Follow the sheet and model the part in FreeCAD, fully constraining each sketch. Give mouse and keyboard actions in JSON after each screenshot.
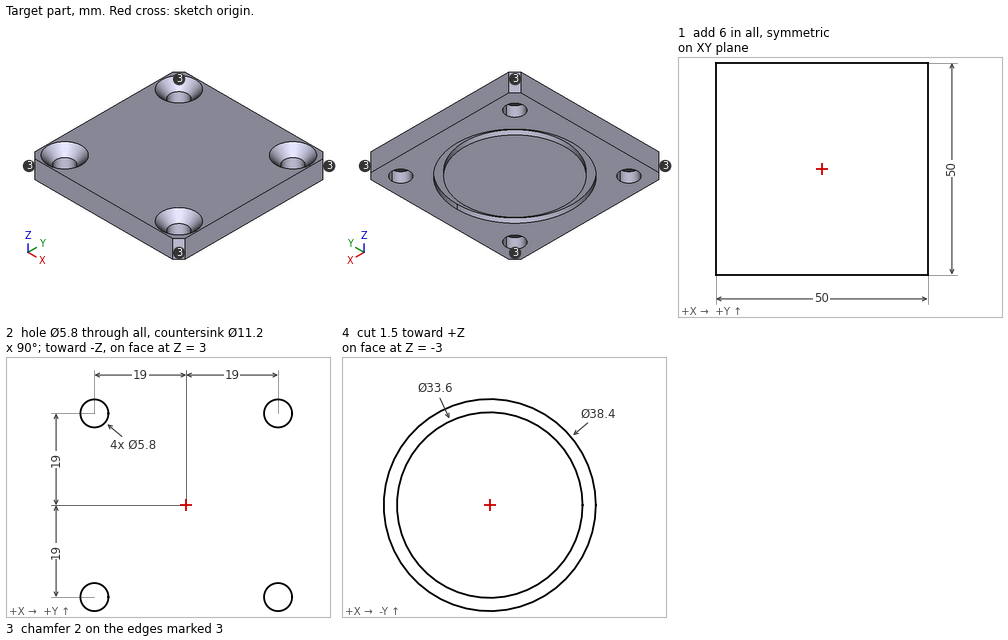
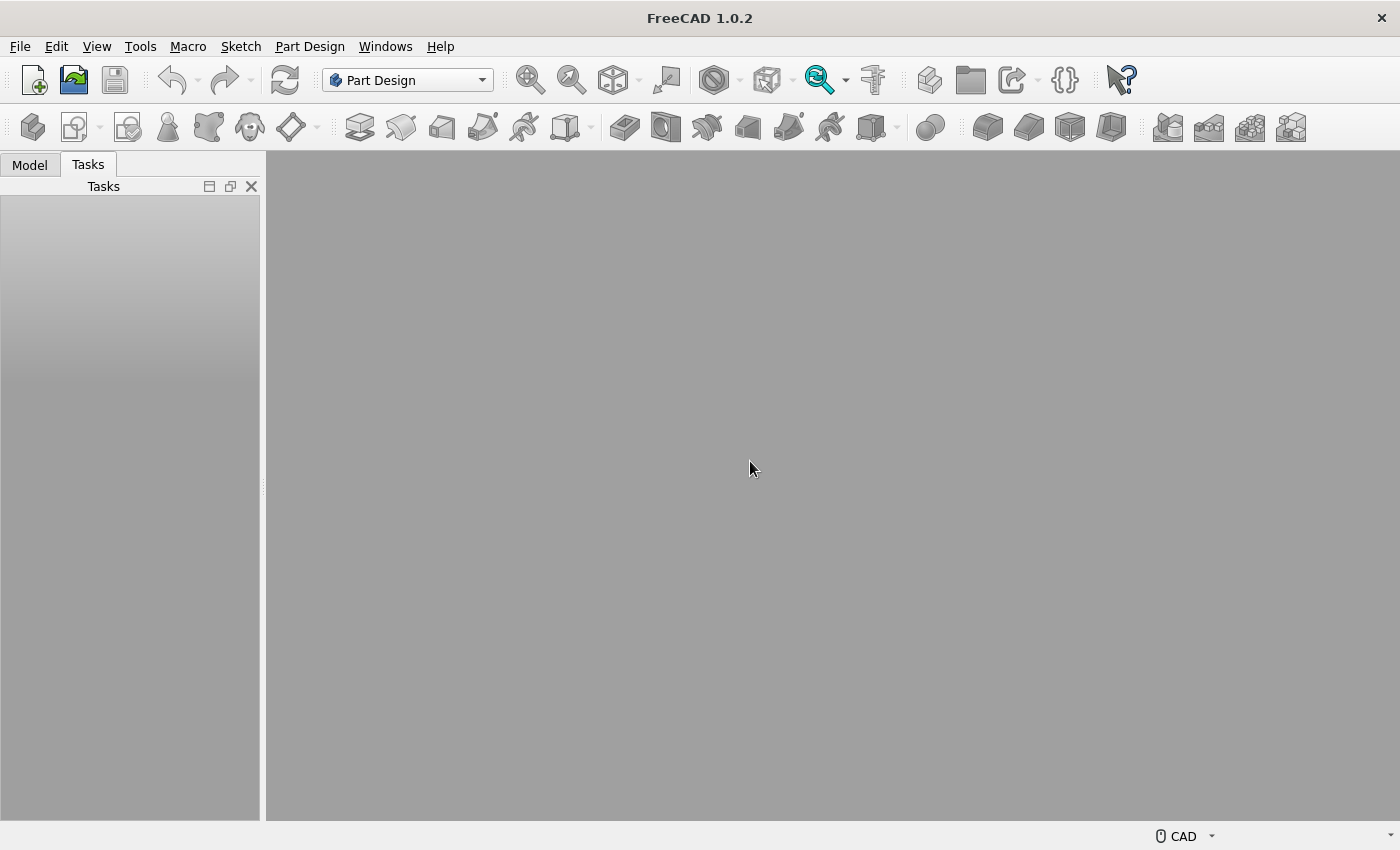
{"action": "left_click", "coordinate": [33, 80]}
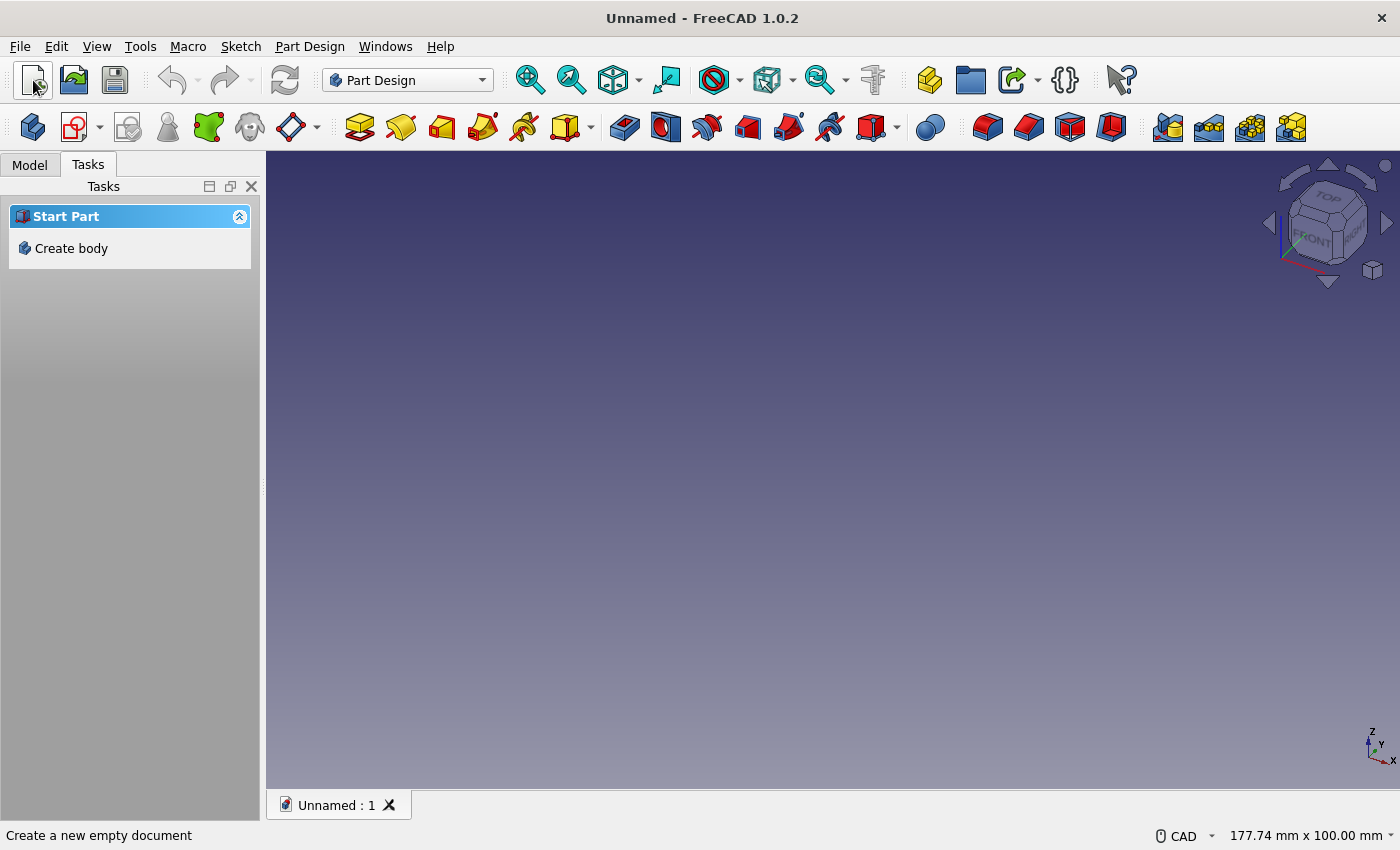
{"action": "left_click", "coordinate": [74, 128]}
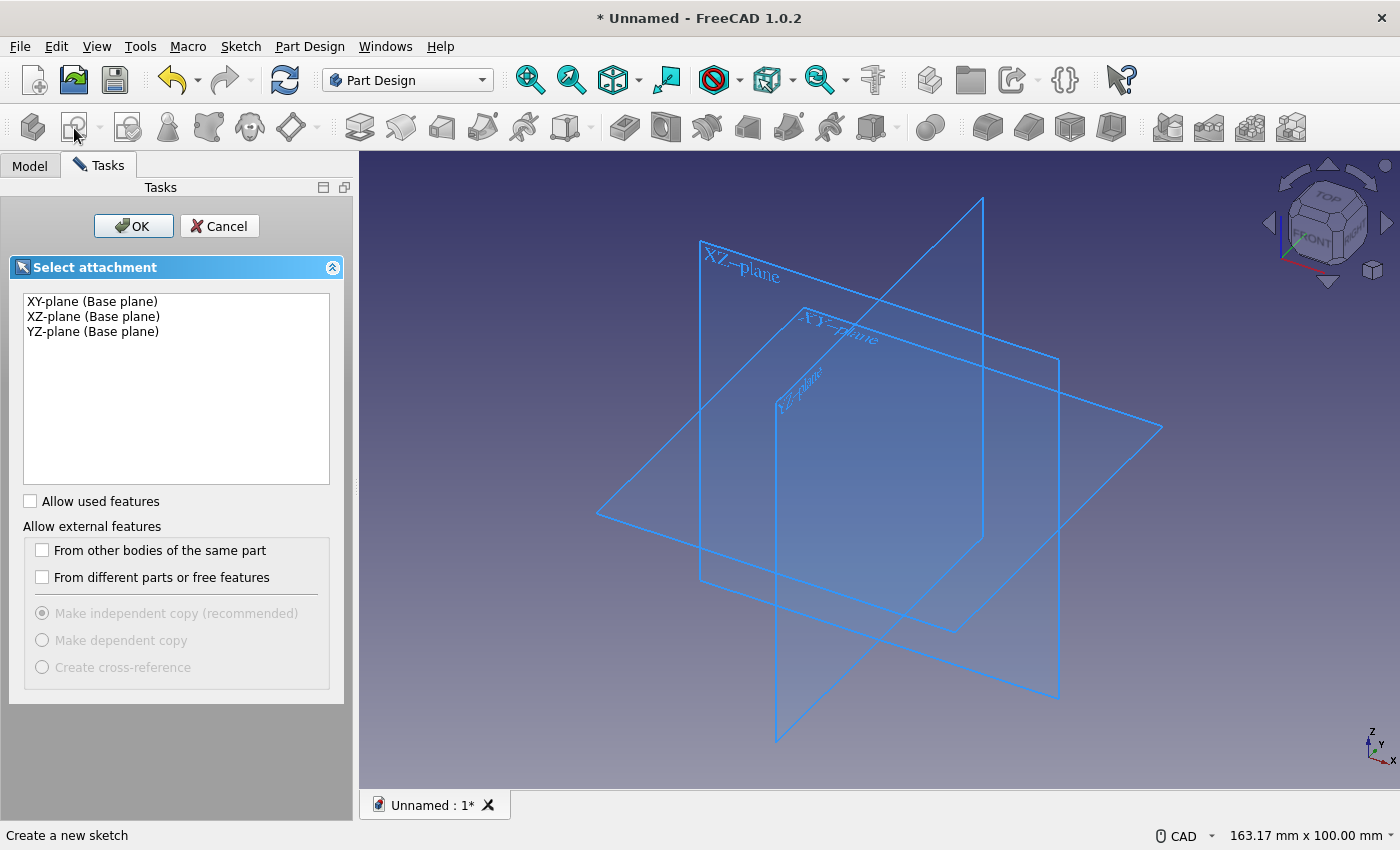
{"action": "left_click", "coordinate": [84, 302]}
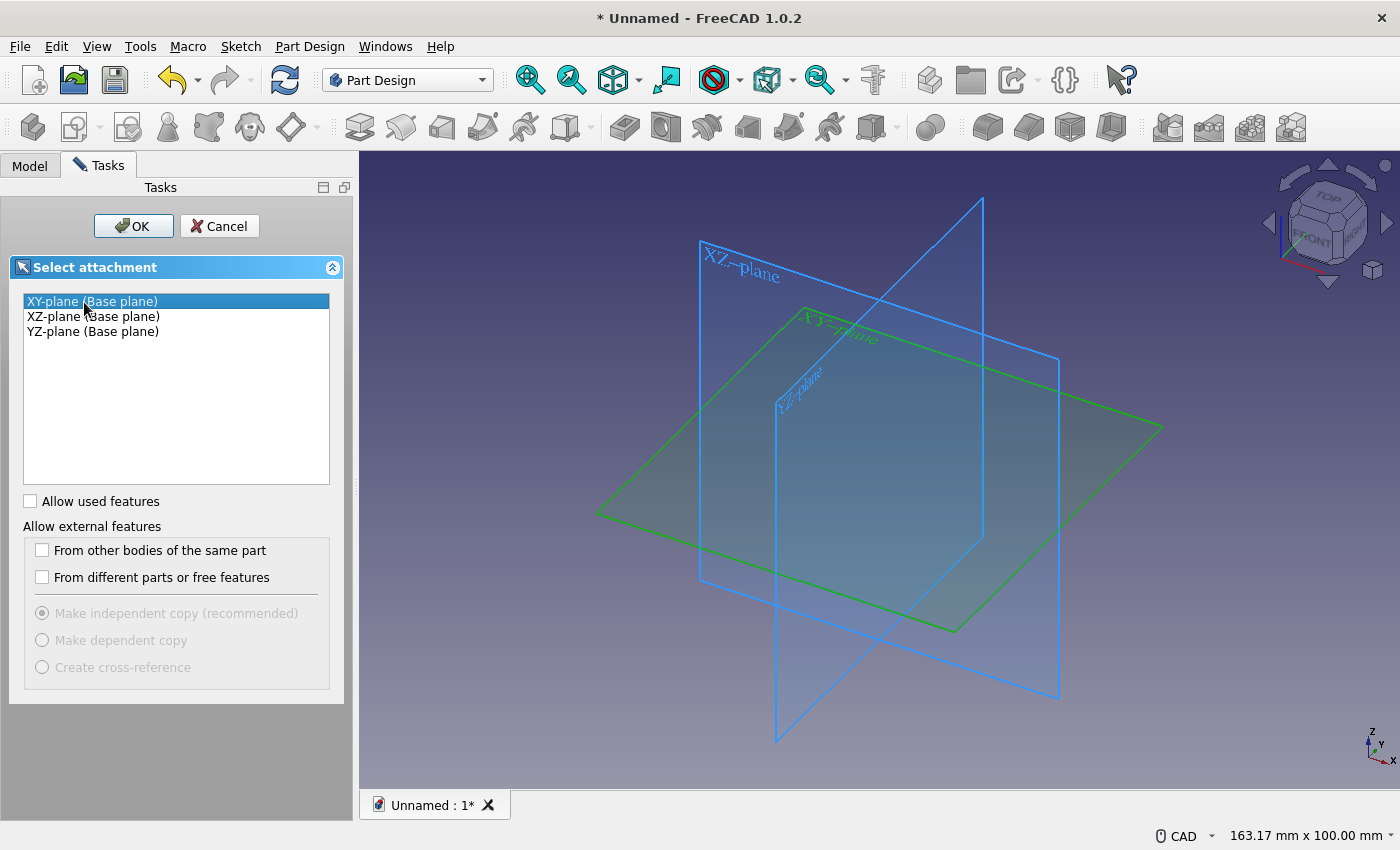
{"action": "left_click", "coordinate": [134, 226]}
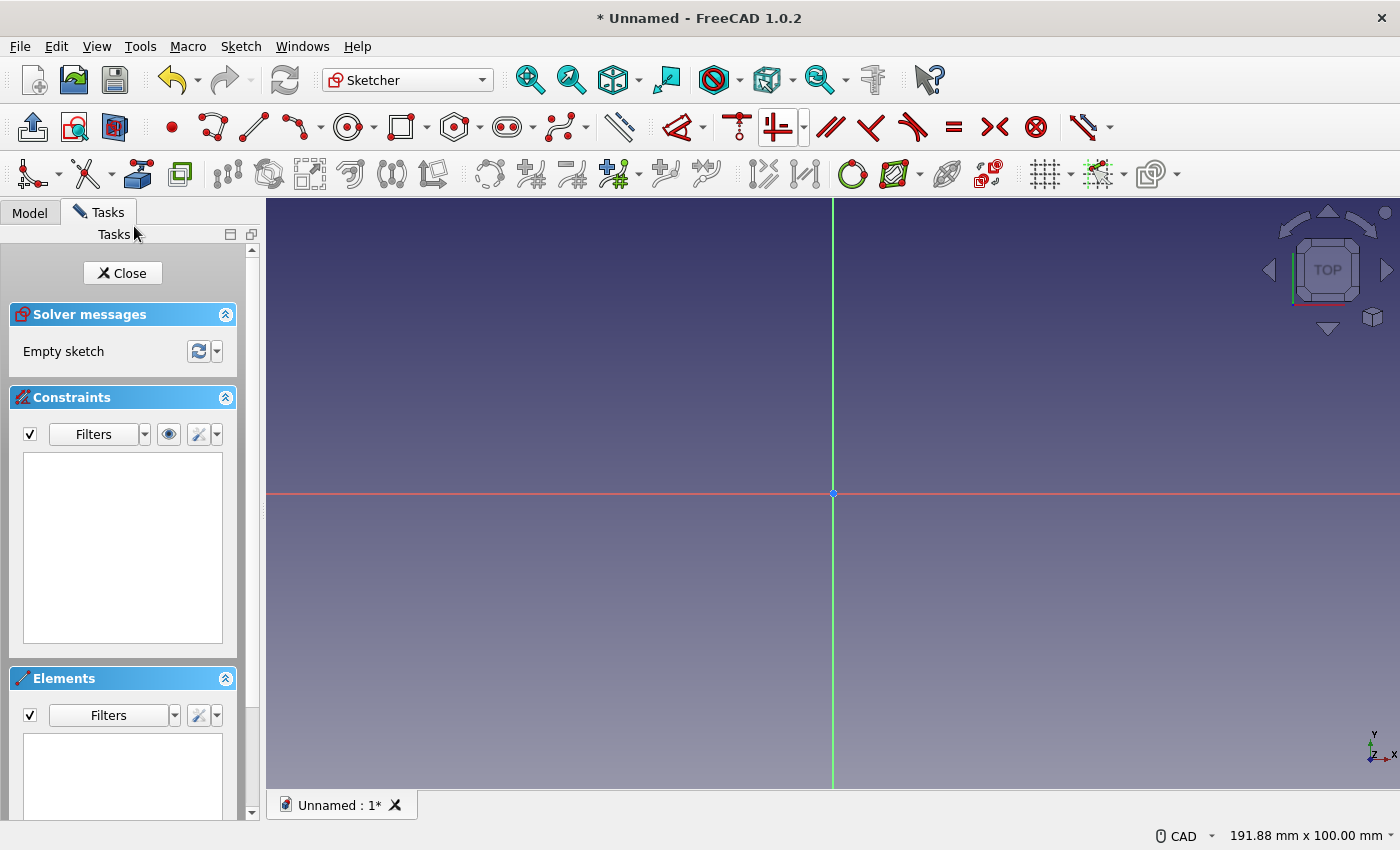
{"action": "left_click", "coordinate": [426, 128]}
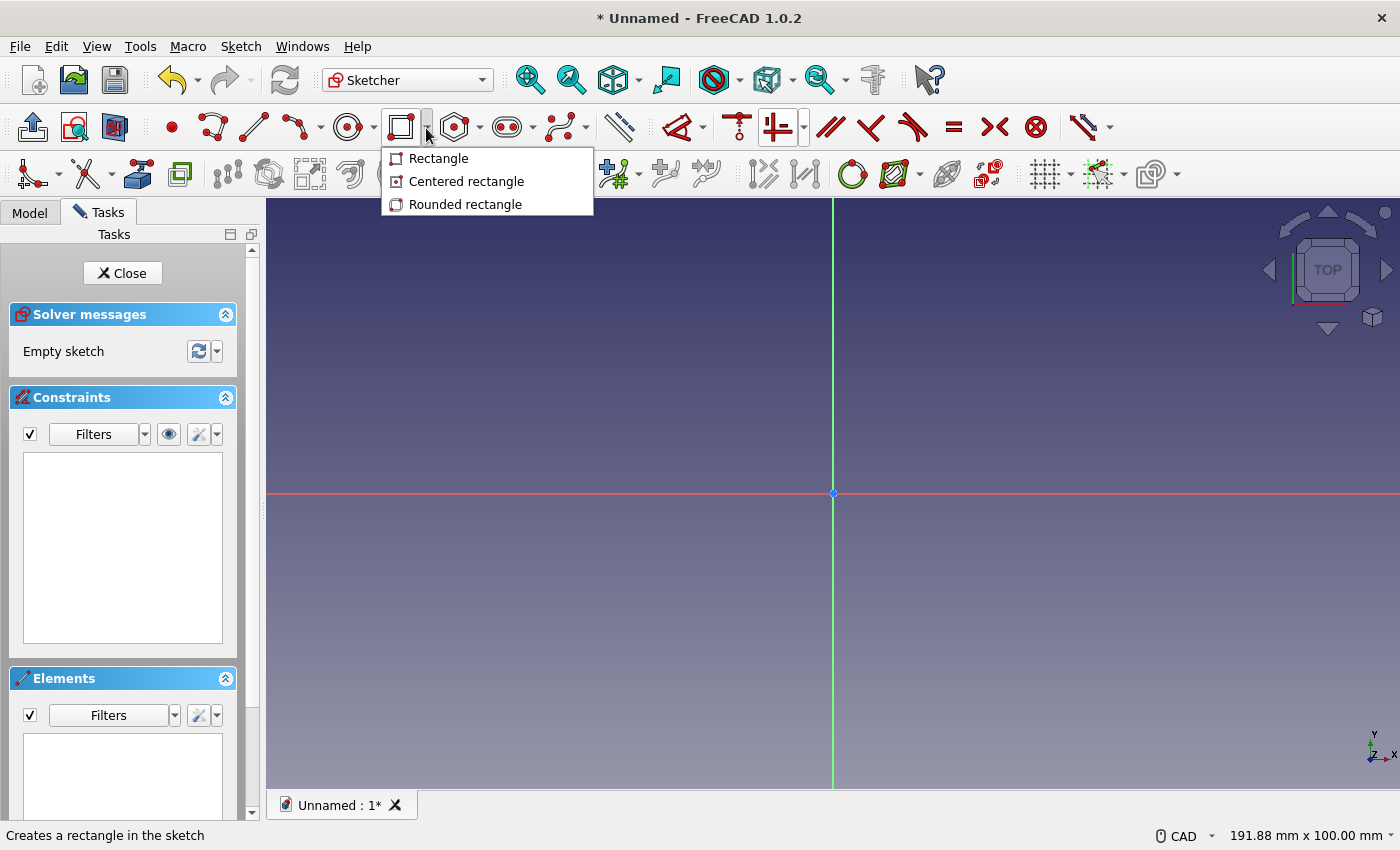
{"action": "left_click", "coordinate": [488, 182]}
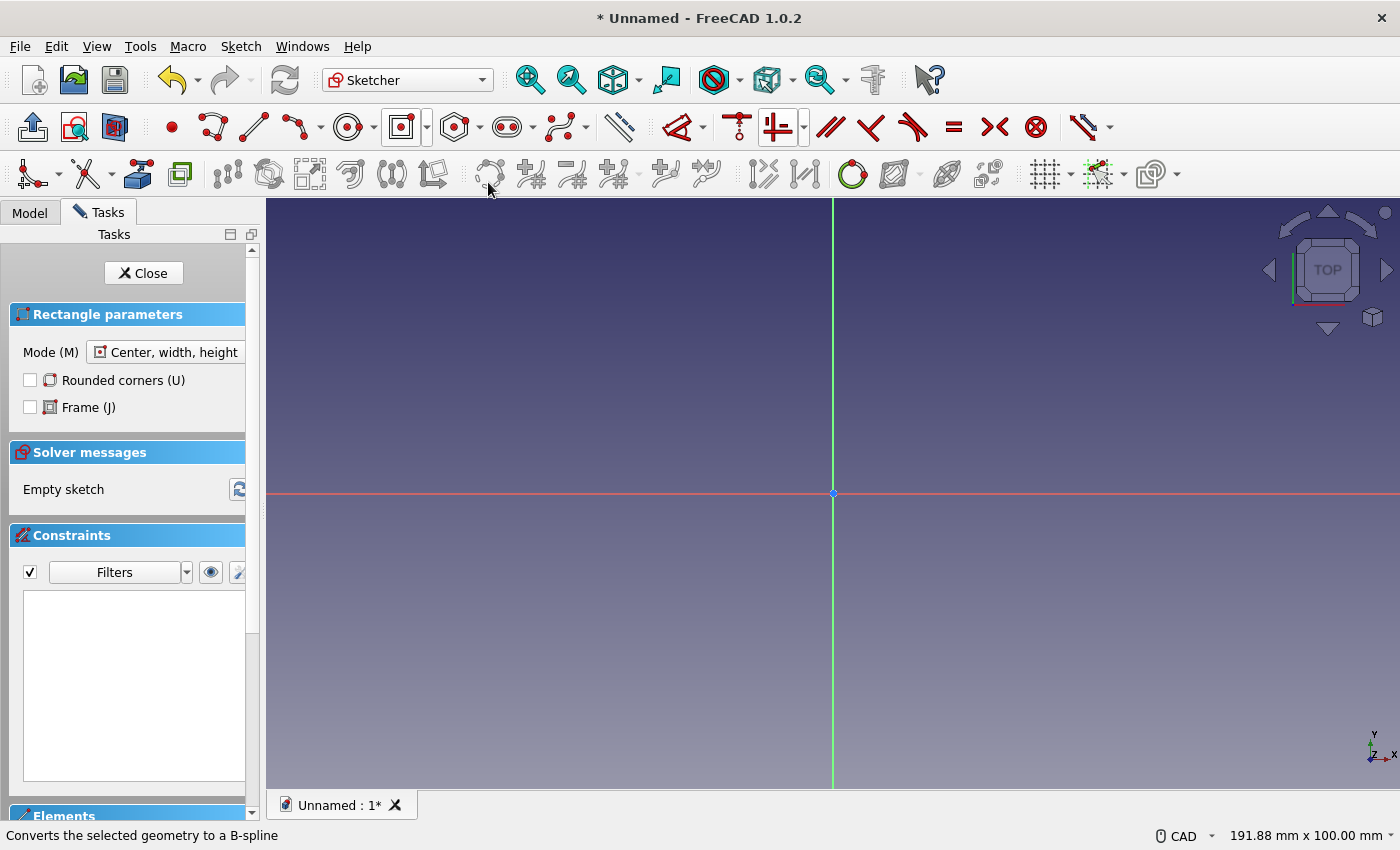
{"action": "left_click", "coordinate": [833, 494]}
{"action": "left_click", "coordinate": [981, 346]}
{"action": "key", "text": "Escape"}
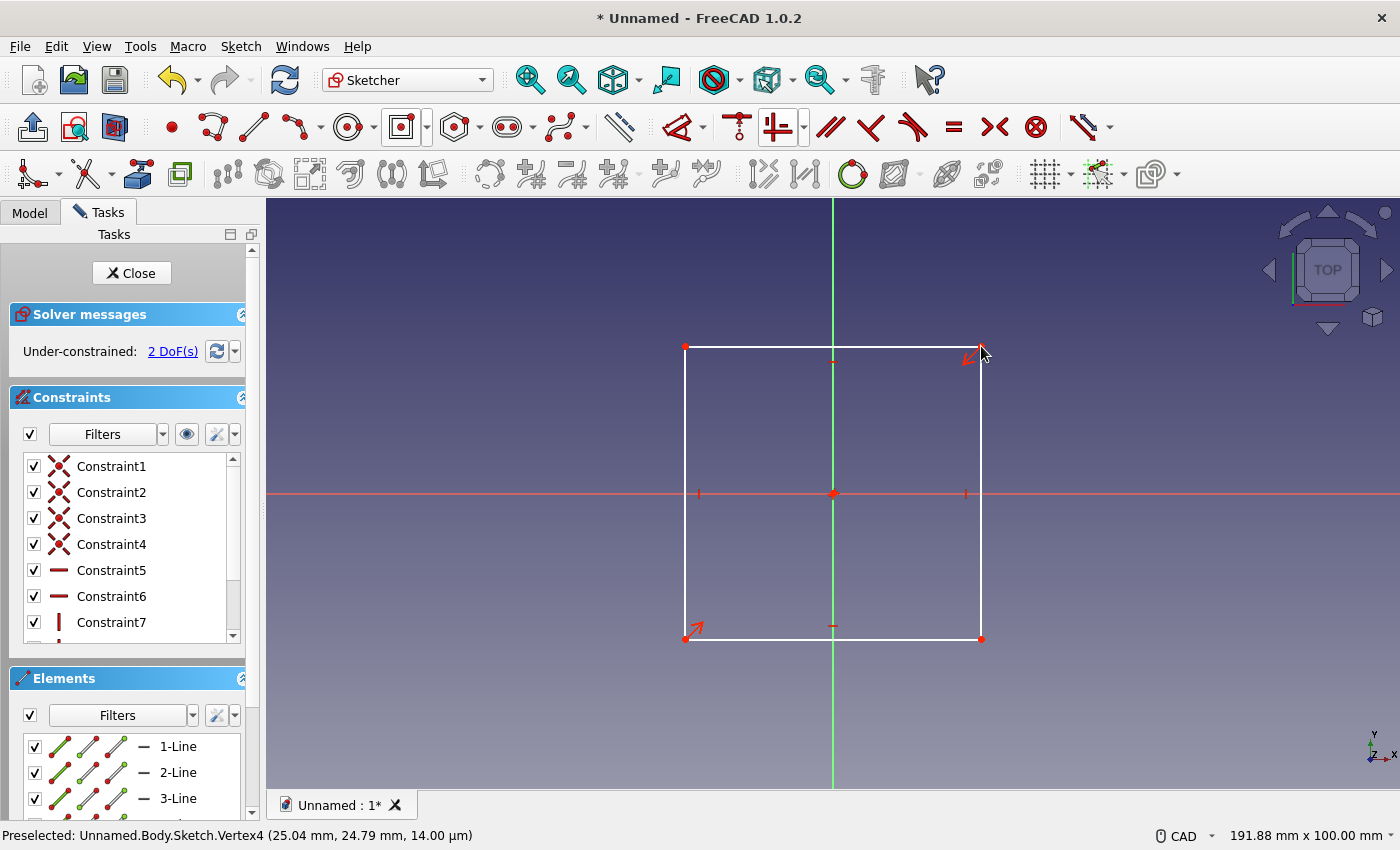
{"action": "left_click", "coordinate": [774, 640]}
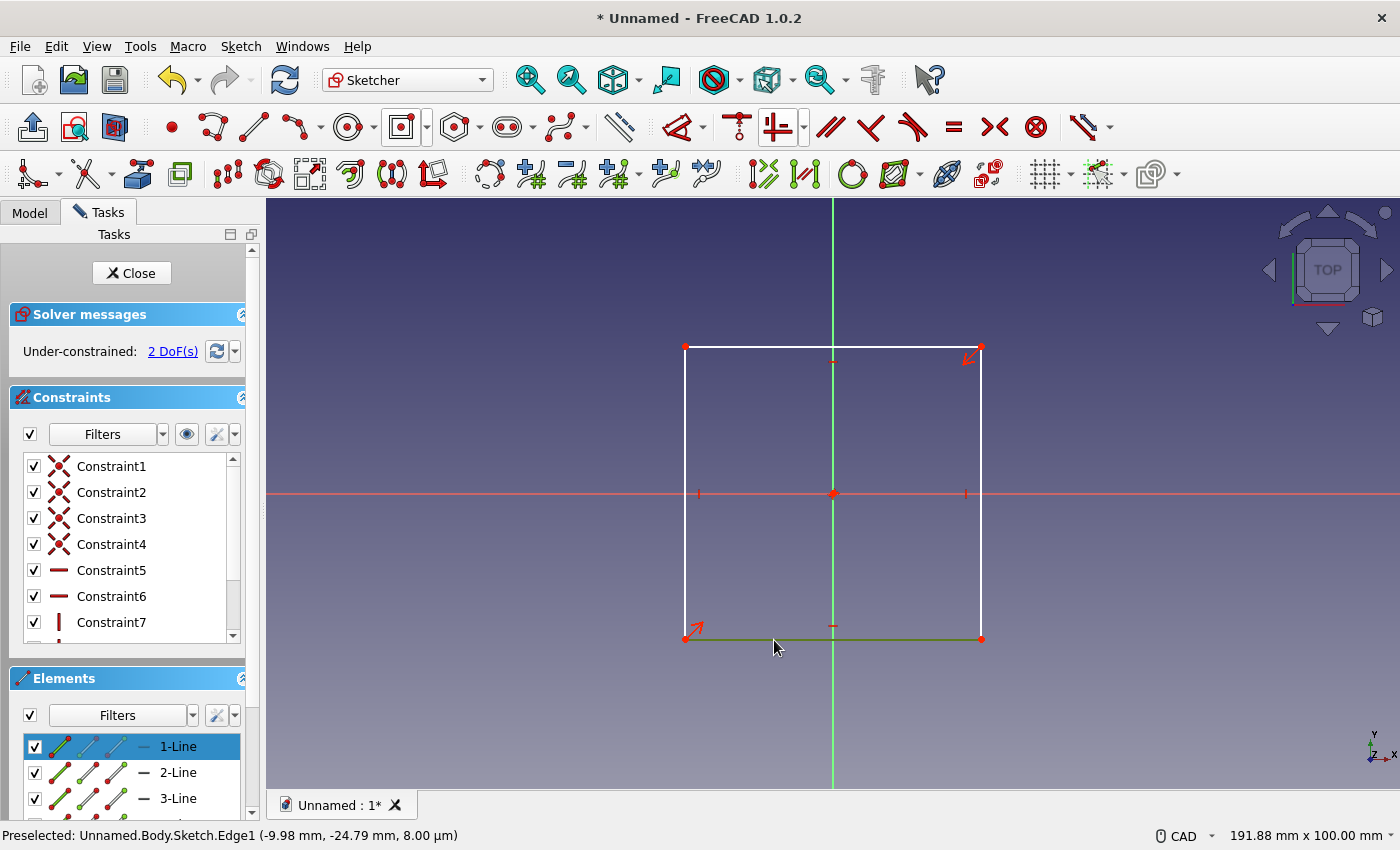
{"action": "key", "text": "l"}